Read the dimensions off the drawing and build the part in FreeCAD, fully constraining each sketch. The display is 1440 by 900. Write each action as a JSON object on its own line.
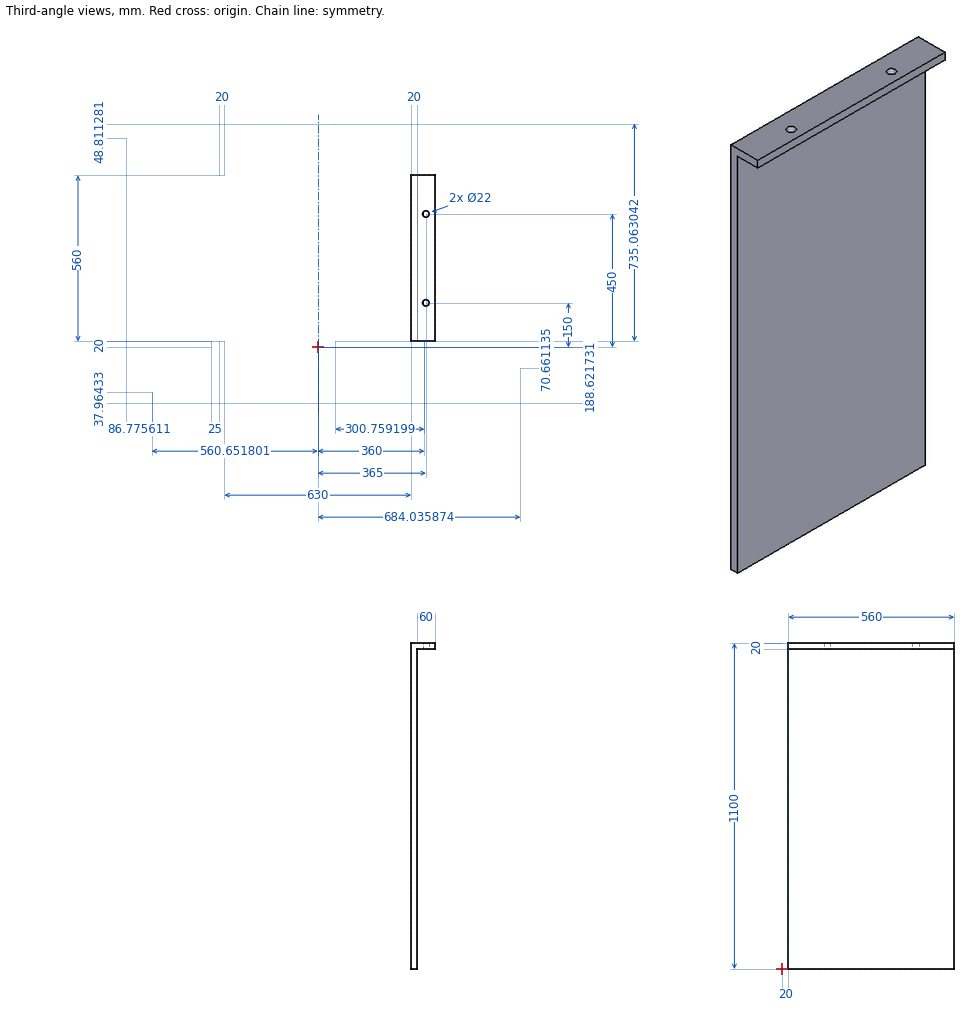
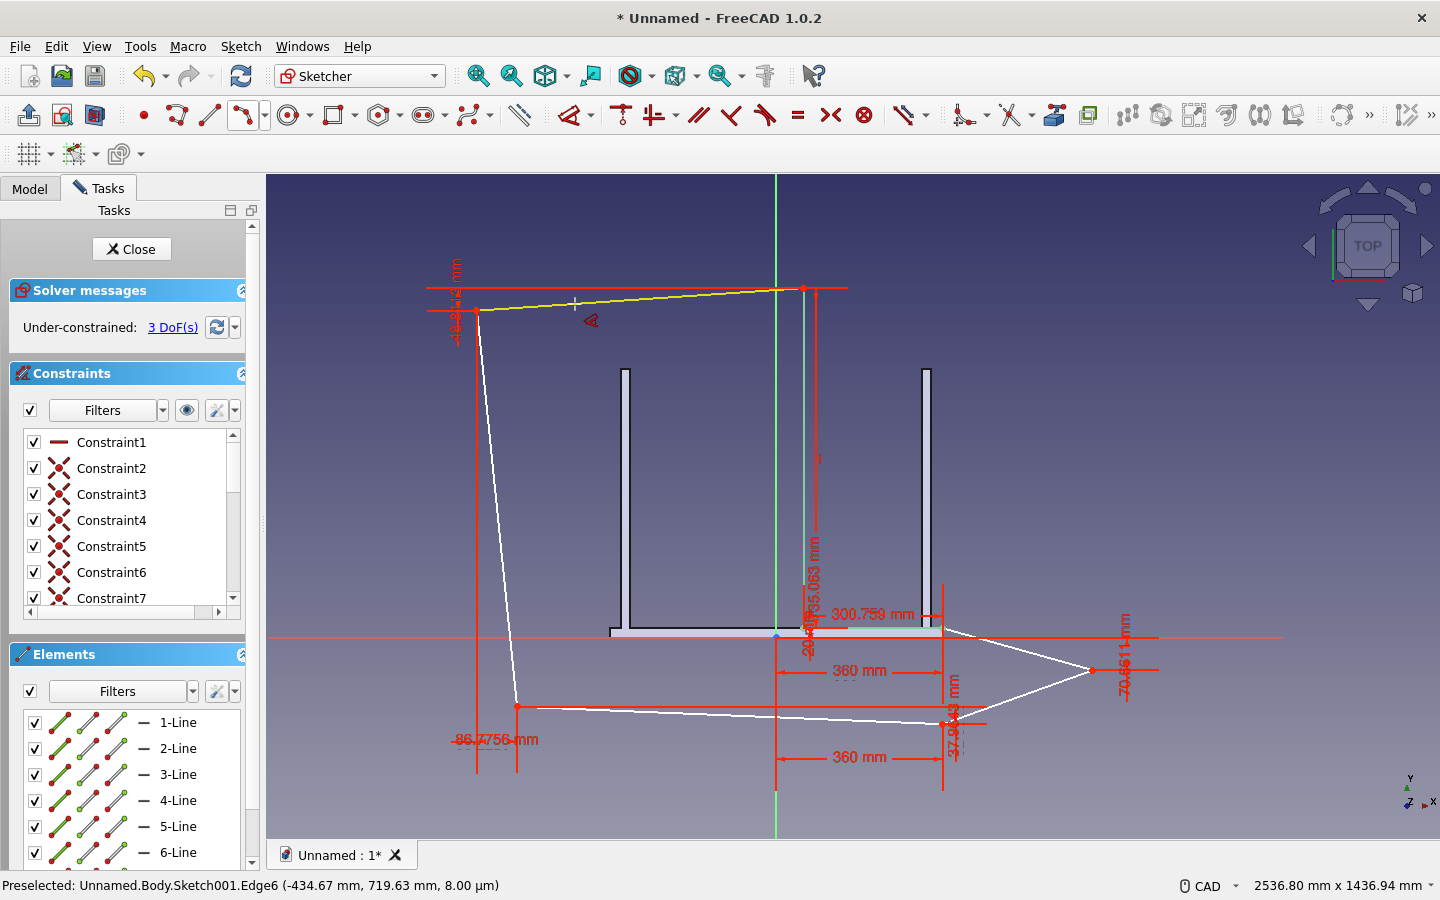
{"action": "left_click", "coordinate": [1093, 670]}
{"action": "left_click", "coordinate": [862, 704]}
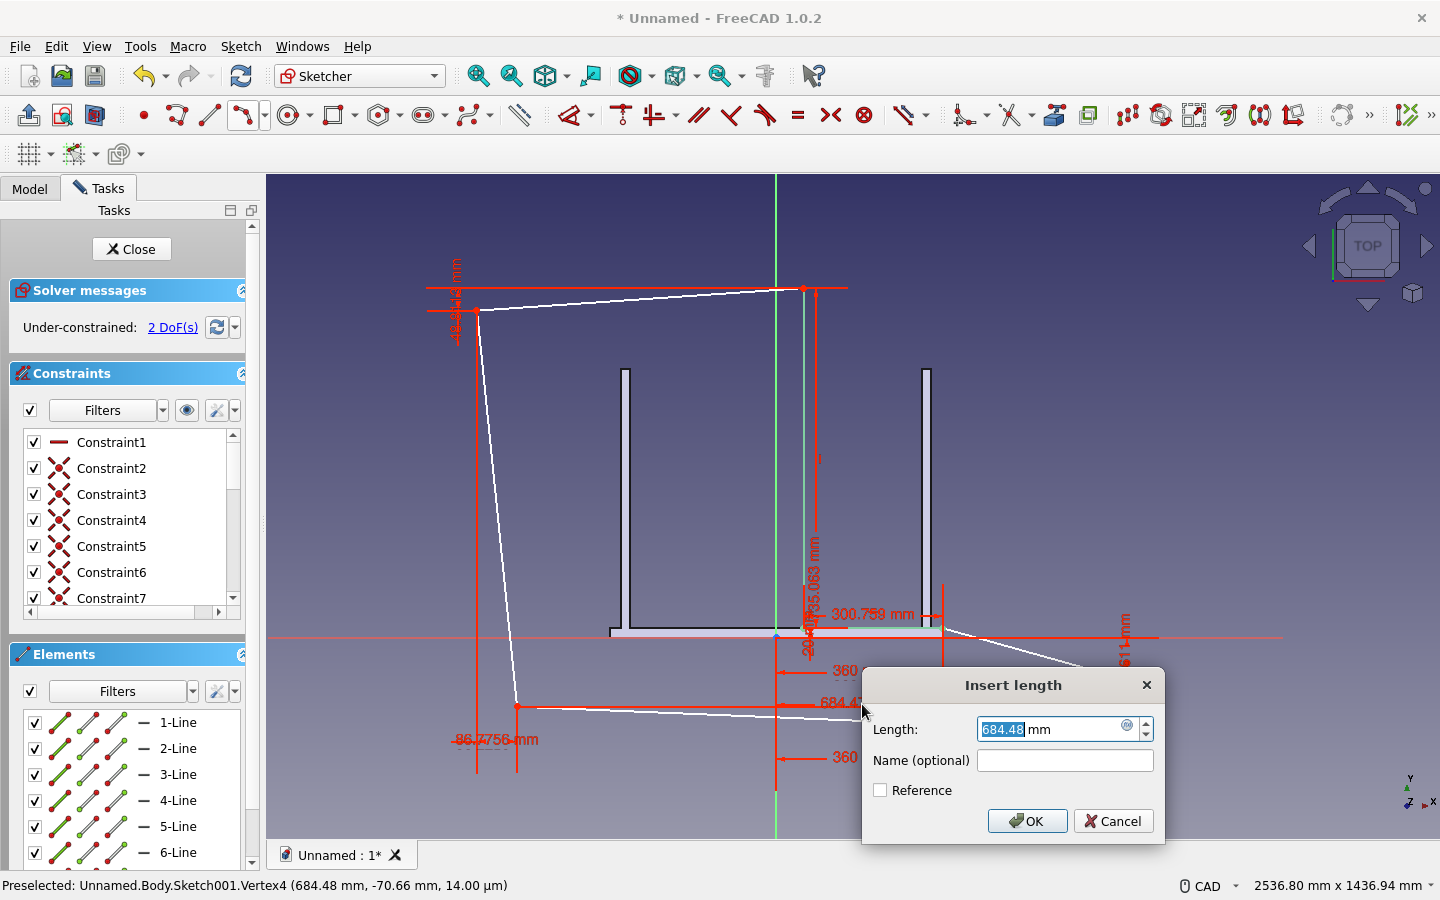
{"action": "type", "text": "684.035874"}
{"action": "key", "text": "Return"}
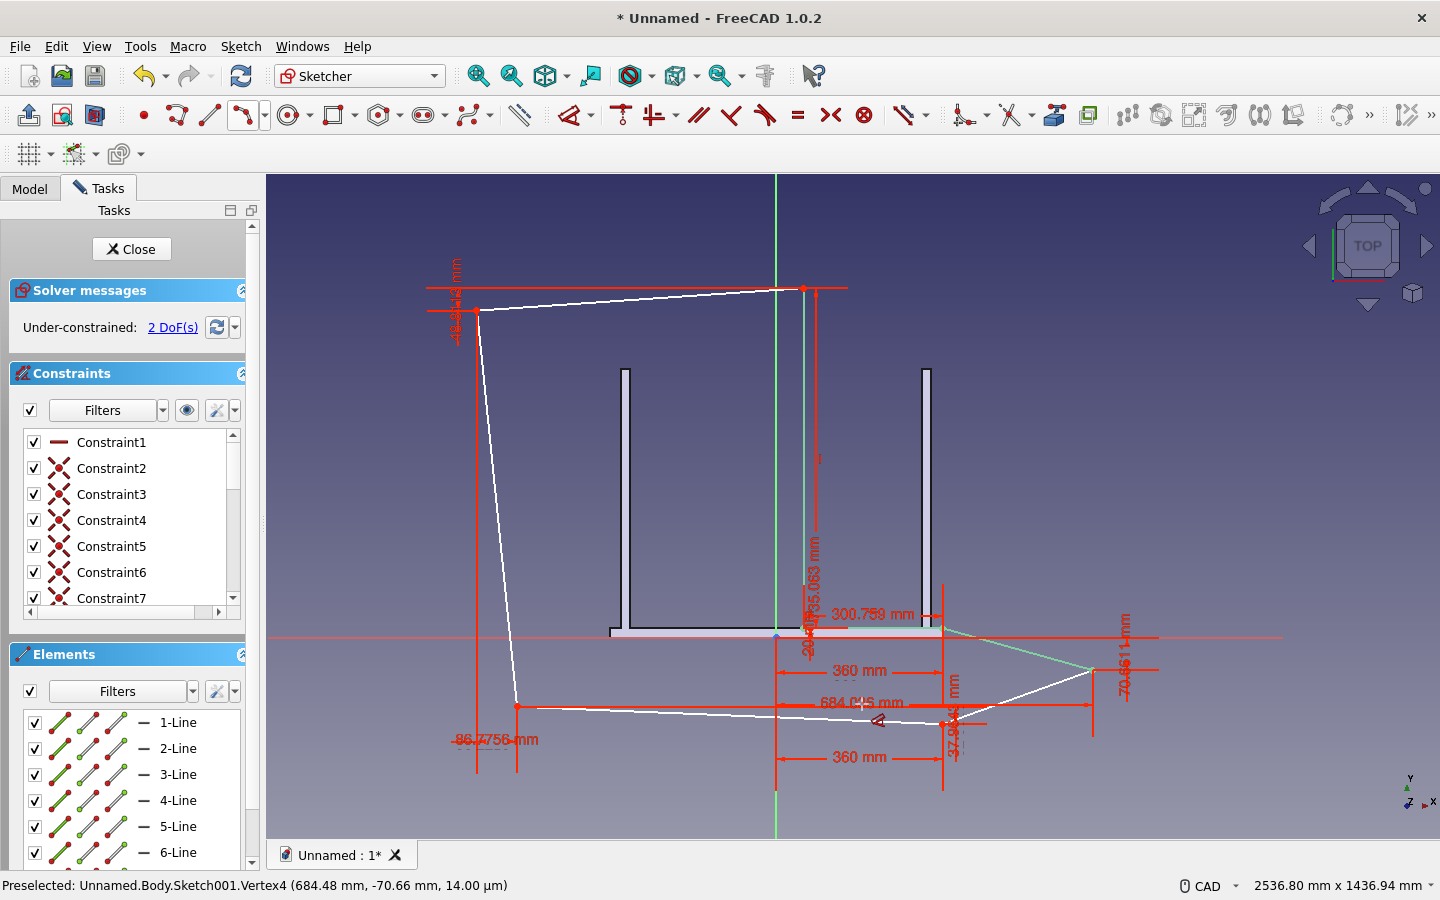
{"action": "left_click", "coordinate": [943, 724]}
{"action": "left_click", "coordinate": [977, 681]}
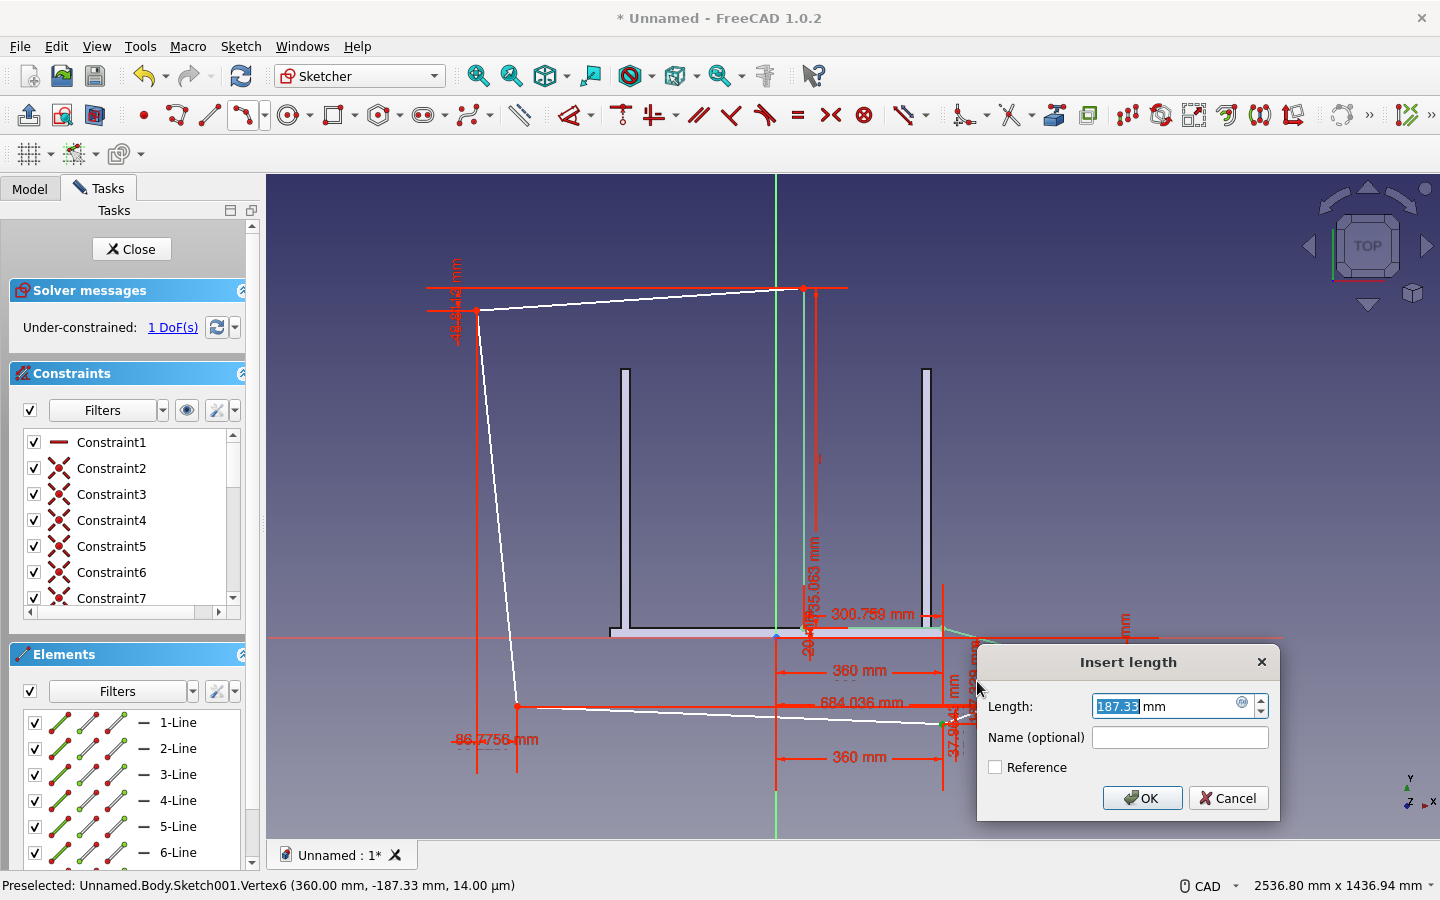
{"action": "type", "text": "188.621731"}
{"action": "key", "text": "Return"}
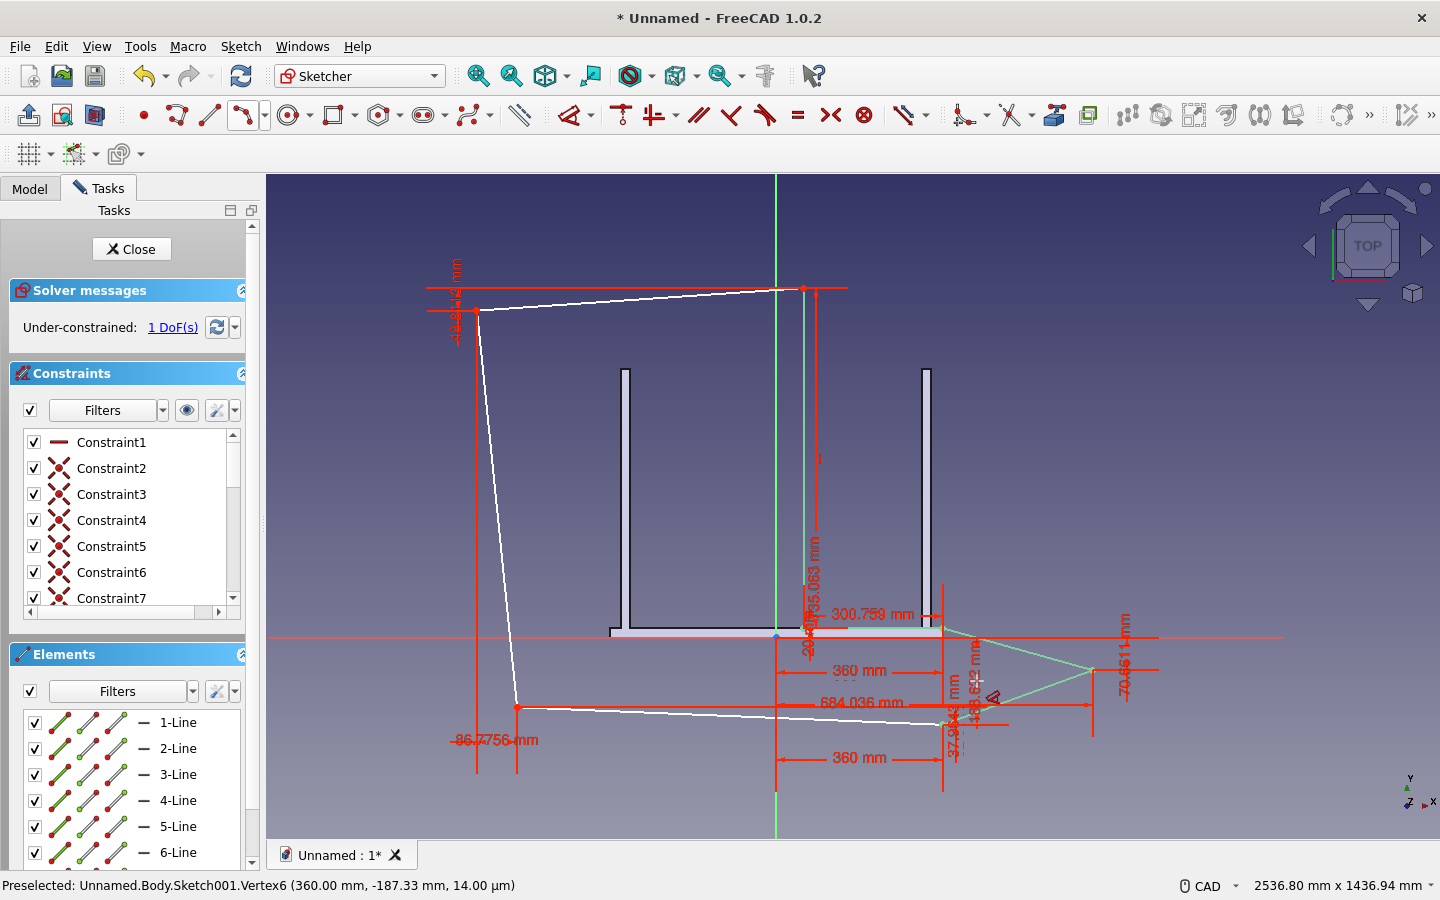
{"action": "left_click", "coordinate": [517, 707]}
{"action": "left_click", "coordinate": [647, 741]}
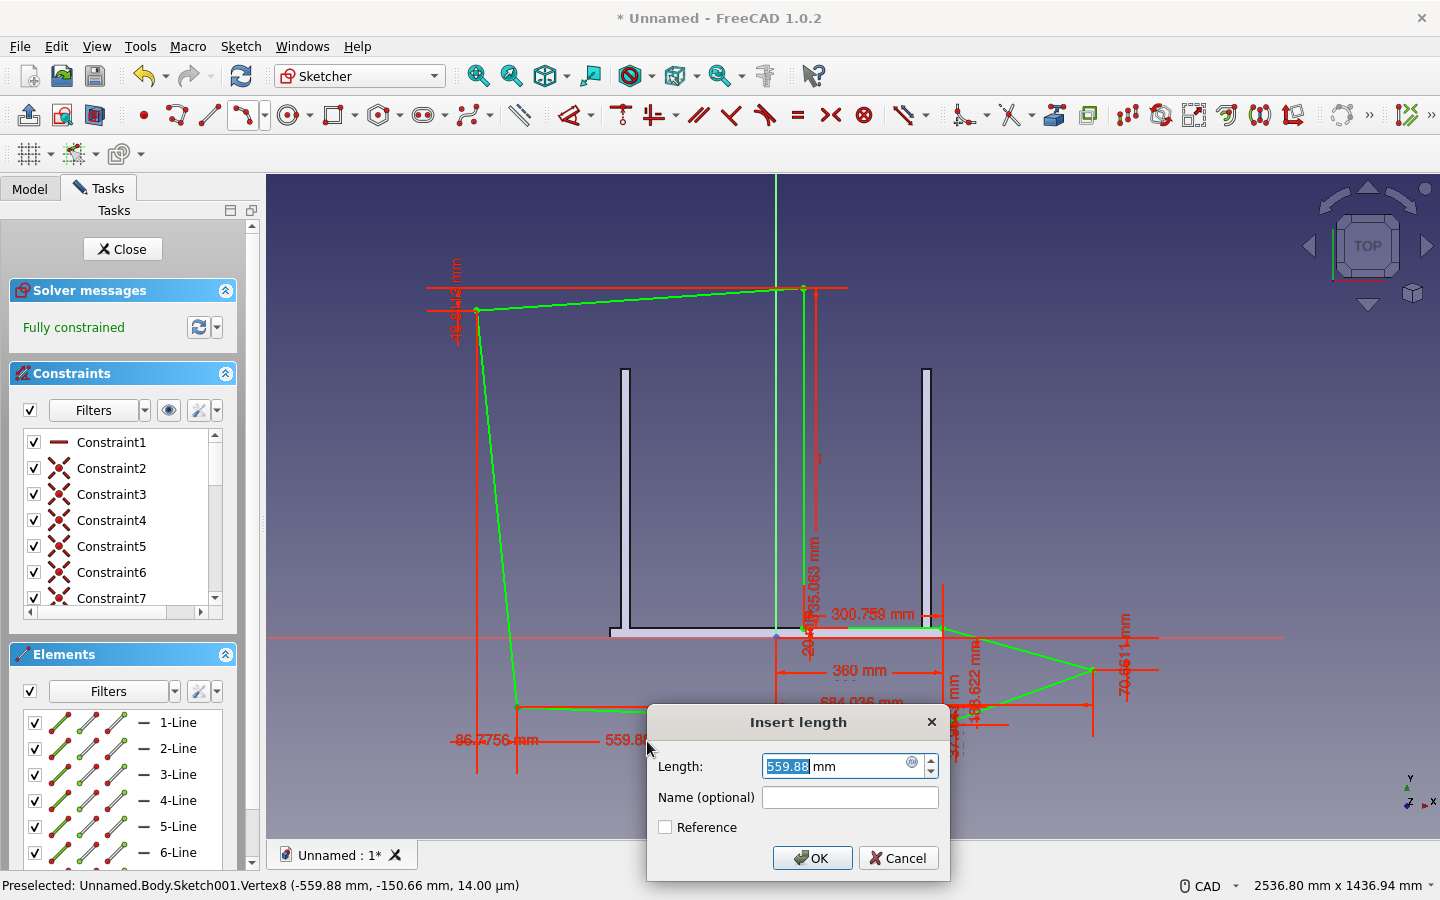
{"action": "type", "text": "560.651801"}
{"action": "key", "text": "Return"}
{"action": "key", "text": "Escape"}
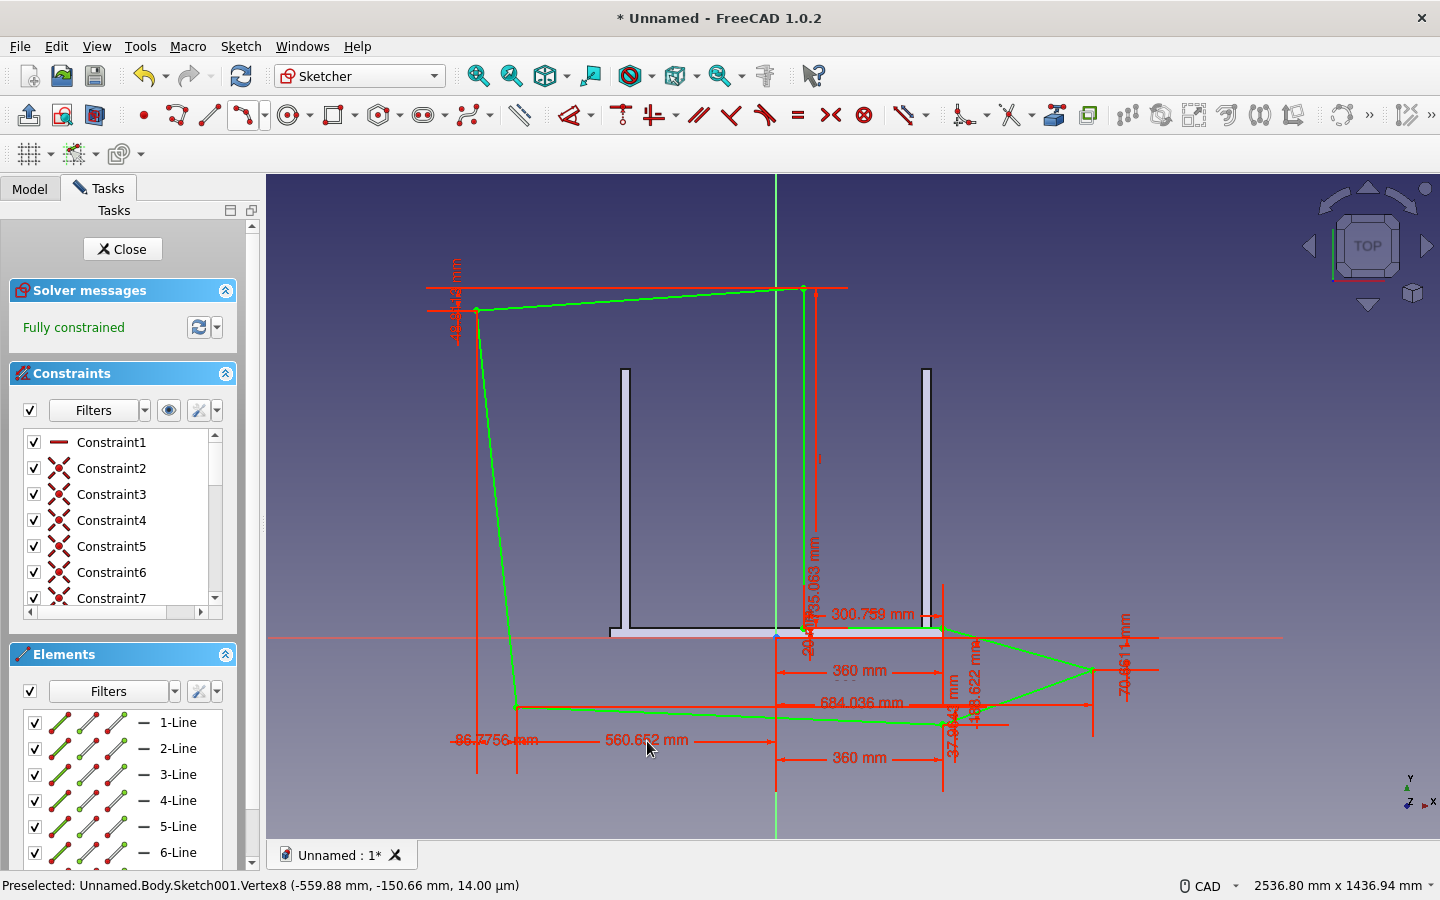
{"action": "left_click", "coordinate": [123, 249]}